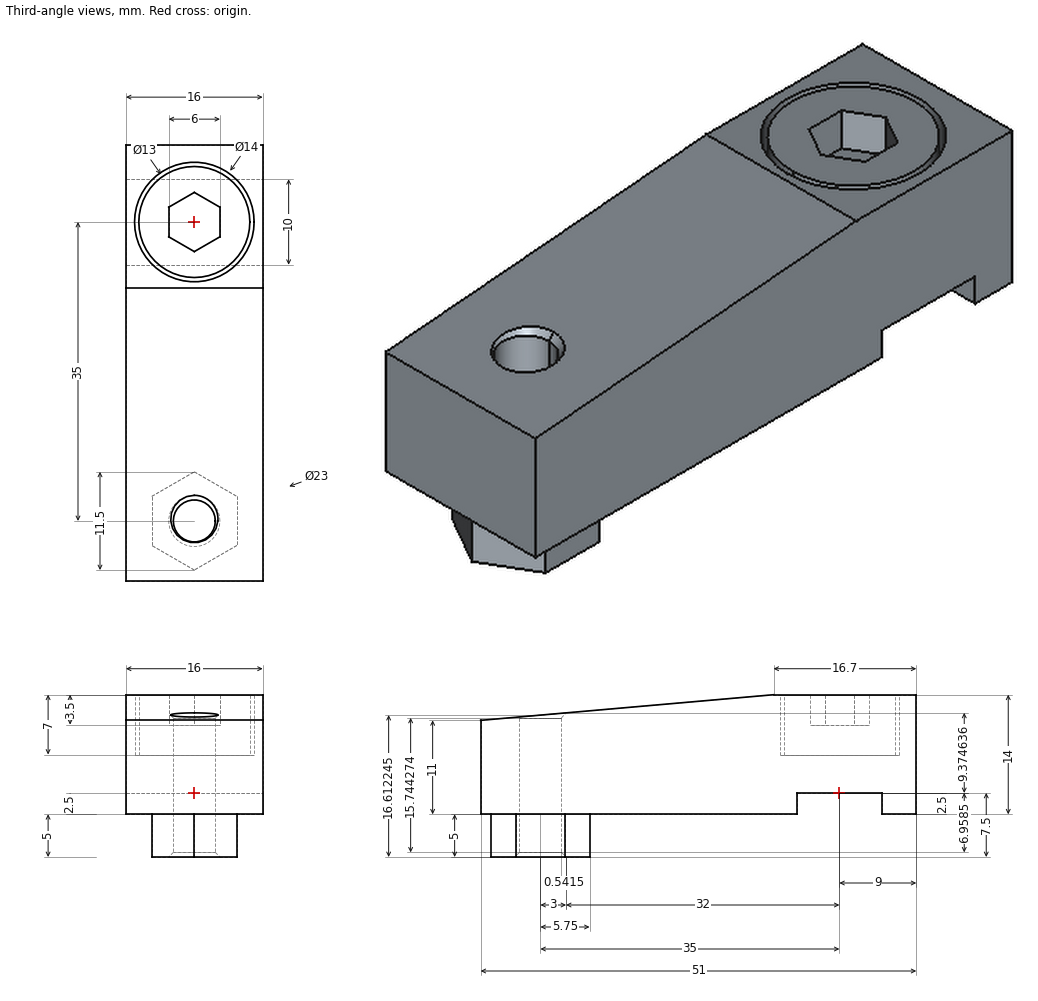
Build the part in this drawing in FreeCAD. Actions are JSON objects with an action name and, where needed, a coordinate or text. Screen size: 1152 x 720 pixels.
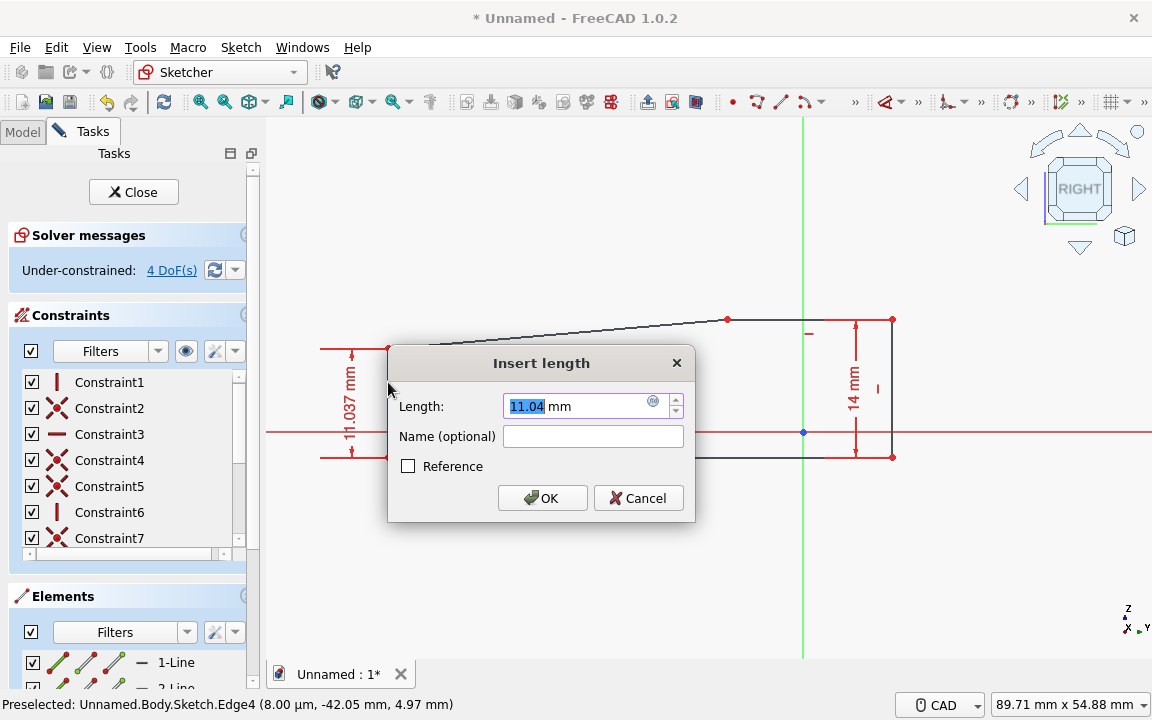
{"action": "type", "text": "11"}
{"action": "key", "text": "Return"}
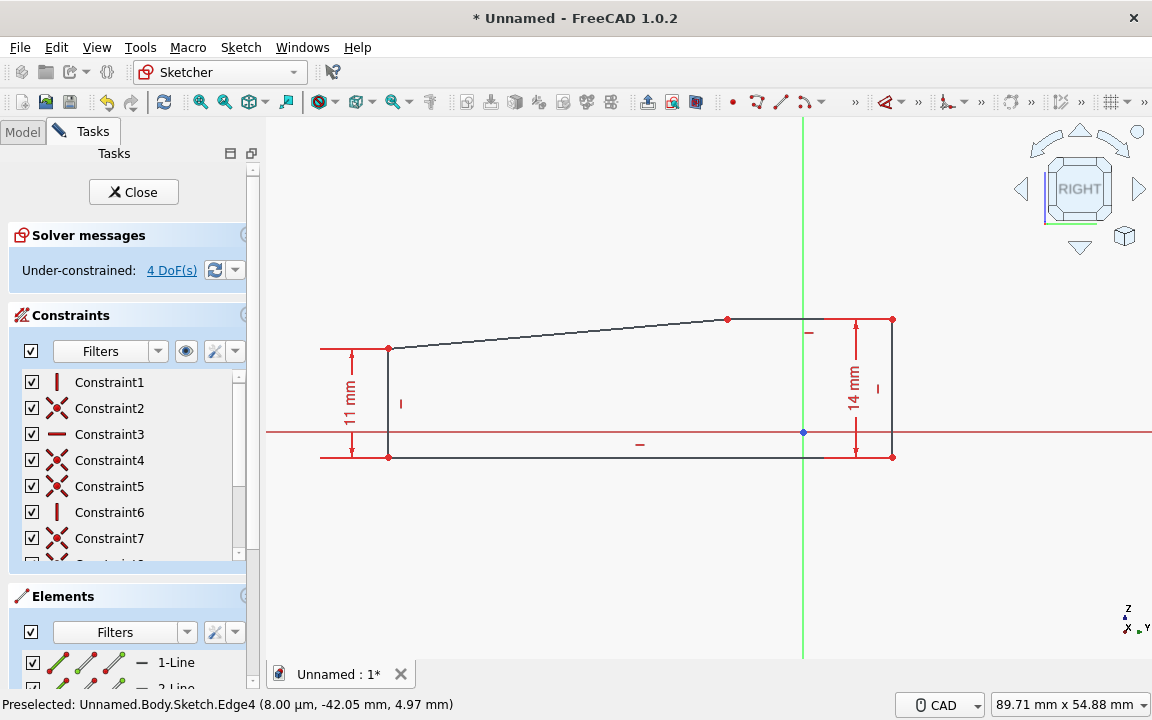
{"action": "left_click", "coordinate": [539, 458]}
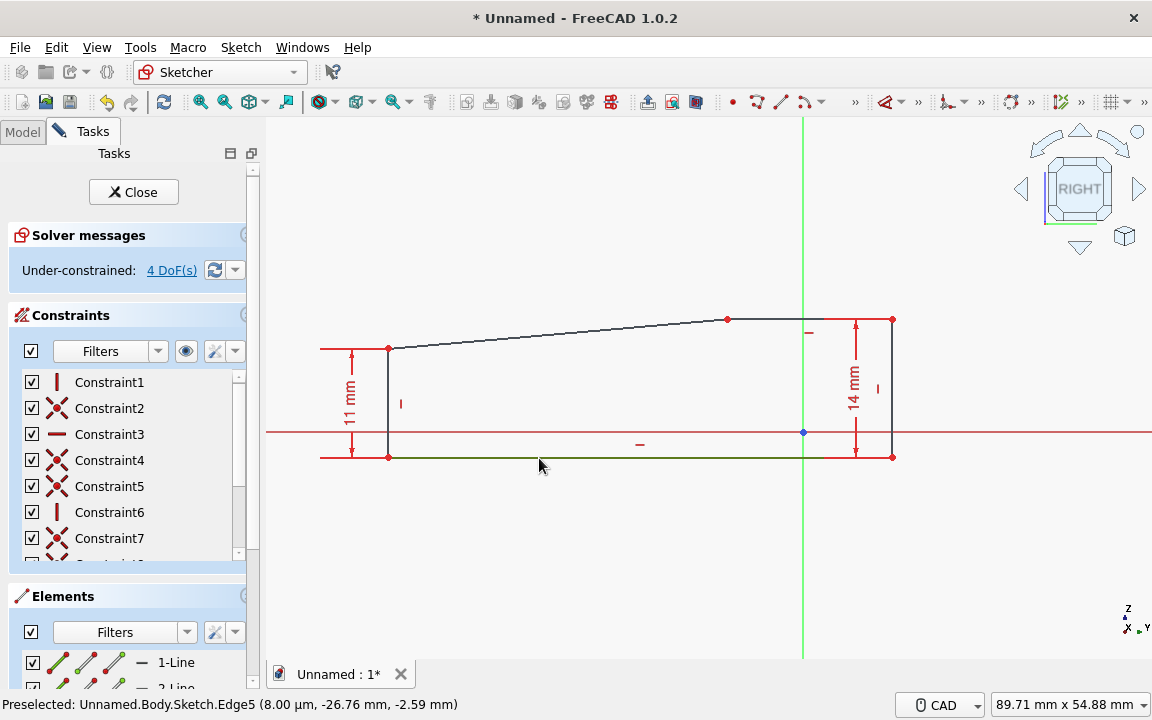
{"action": "left_click", "coordinate": [904, 102]}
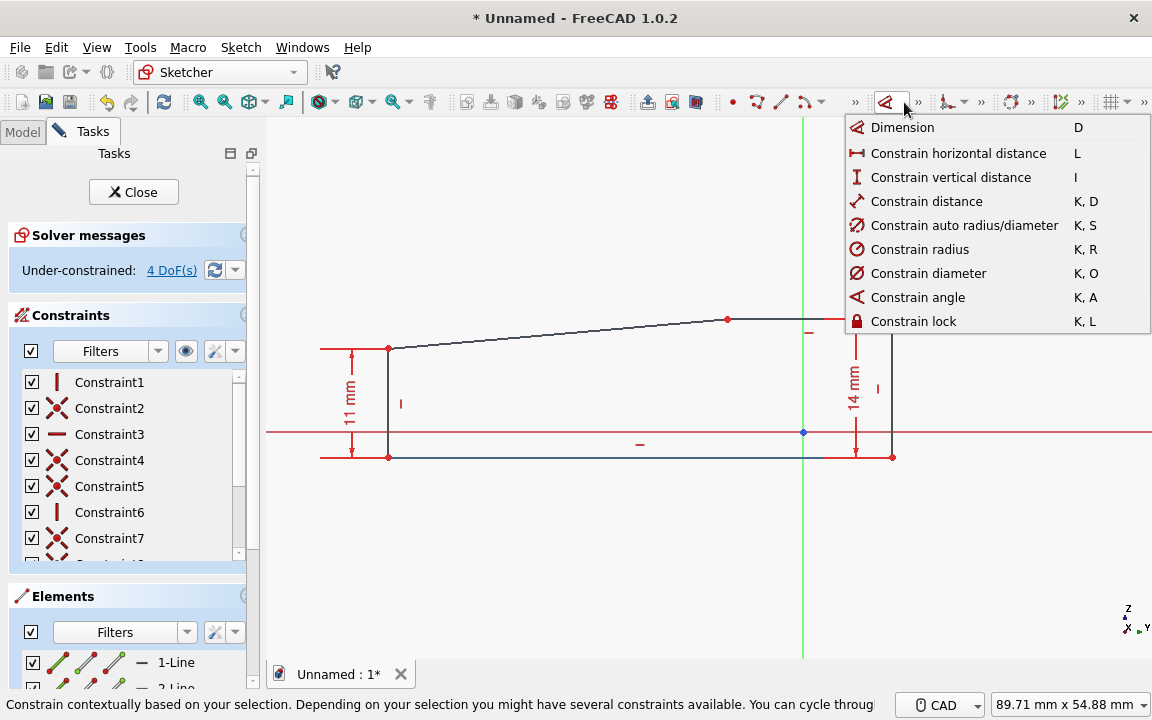
{"action": "left_click", "coordinate": [998, 153]}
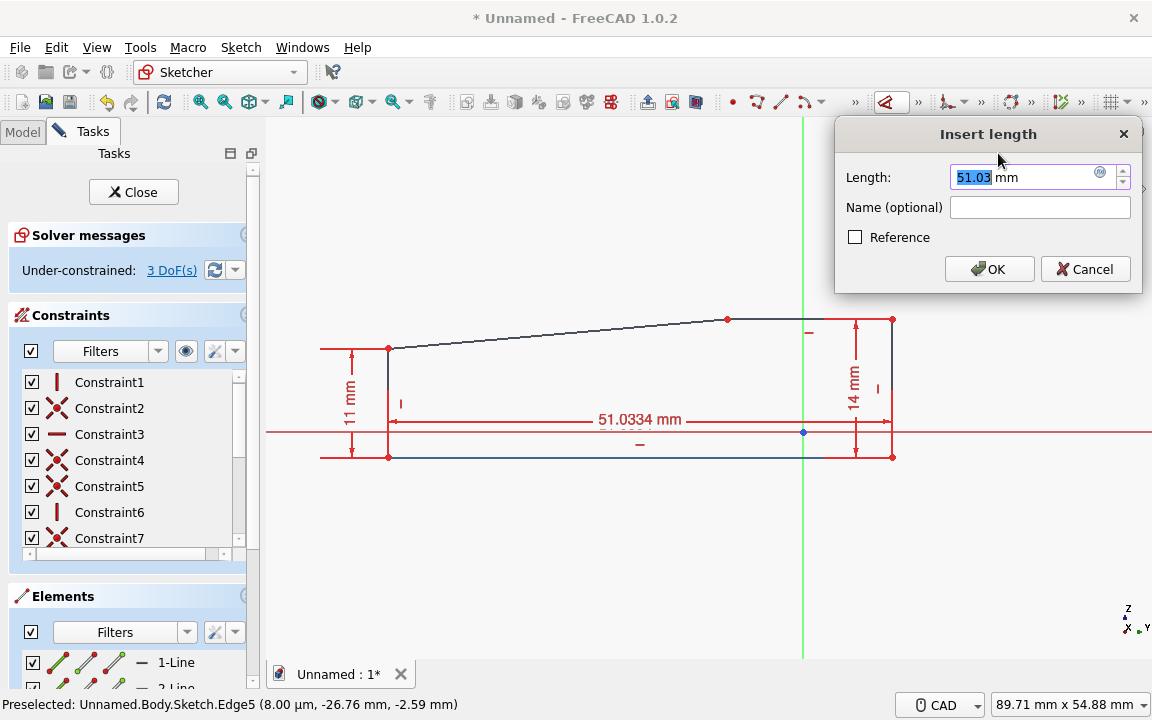
{"action": "type", "text": "51"}
{"action": "key", "text": "Return"}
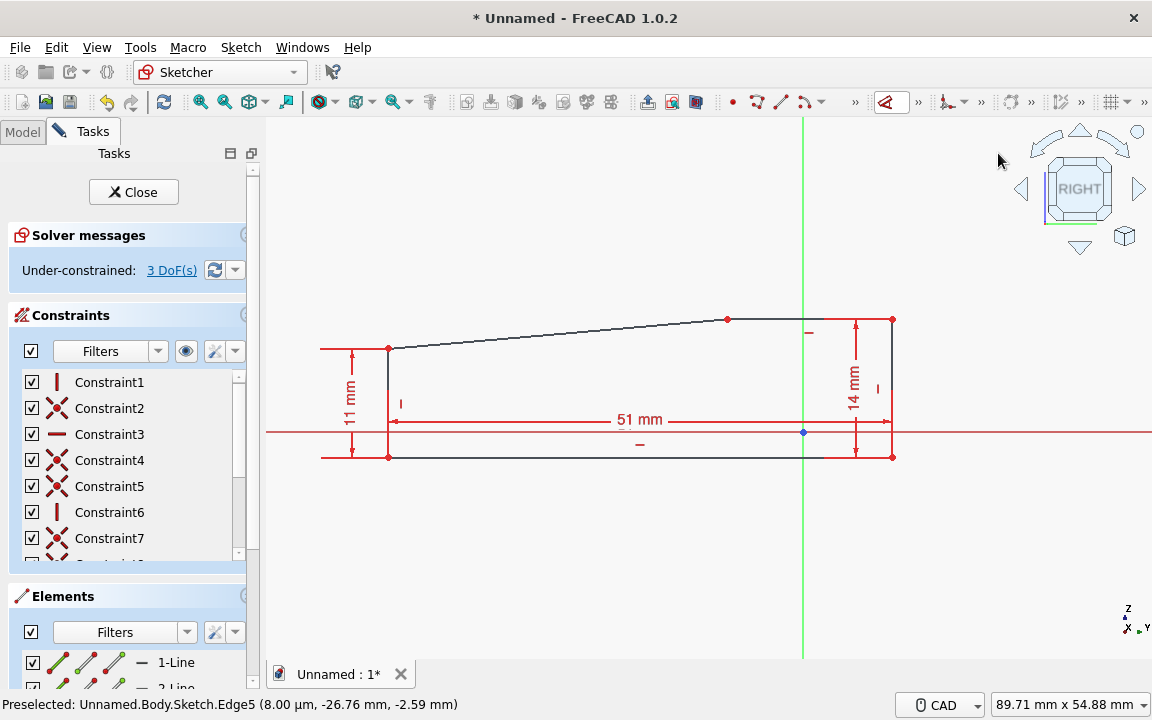
{"action": "left_click", "coordinate": [892, 458]}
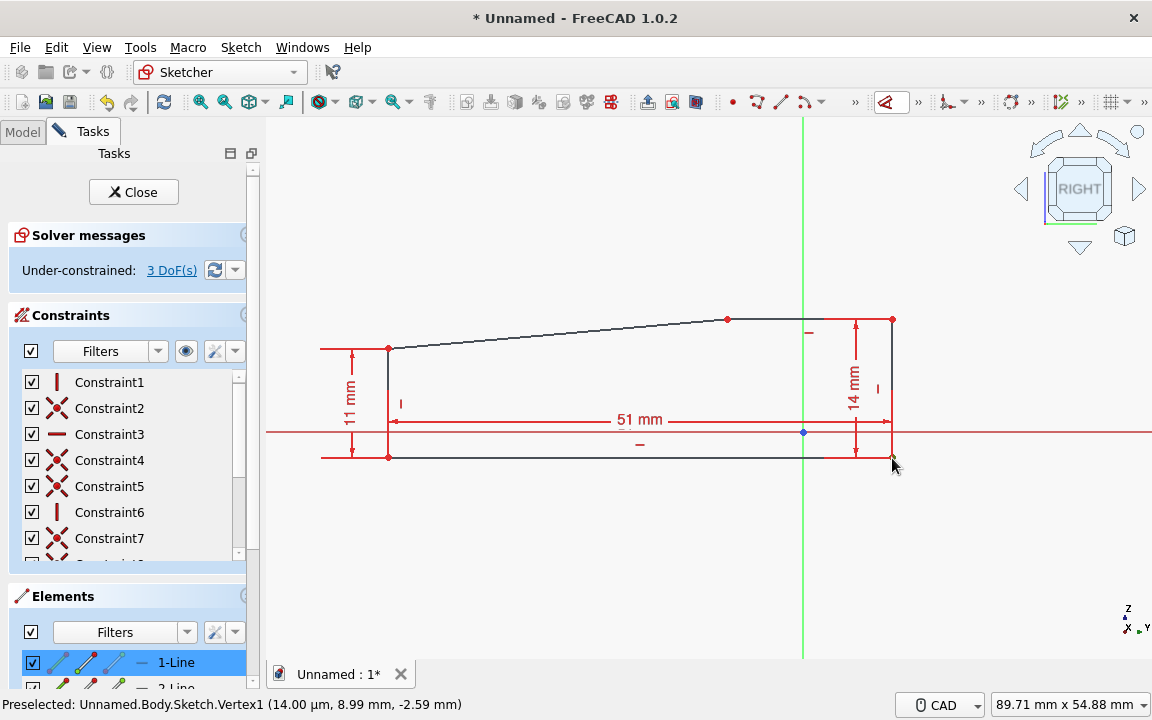
{"action": "key", "text": "l"}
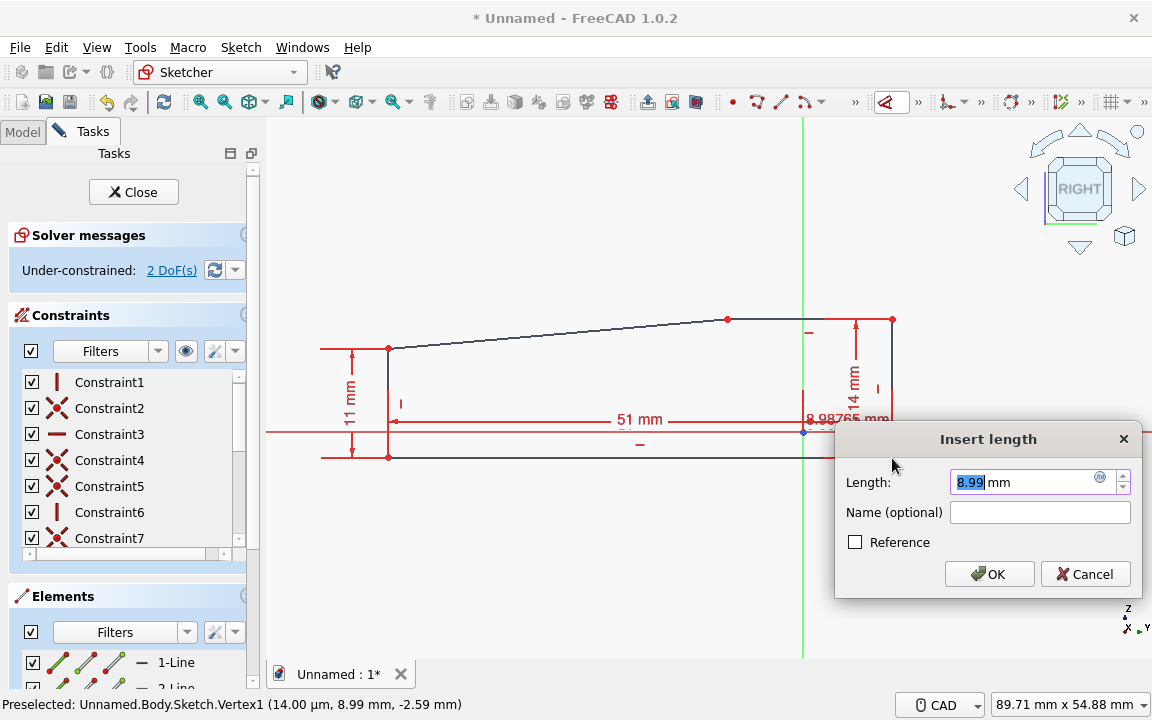
{"action": "type", "text": "9"}
{"action": "key", "text": "Return"}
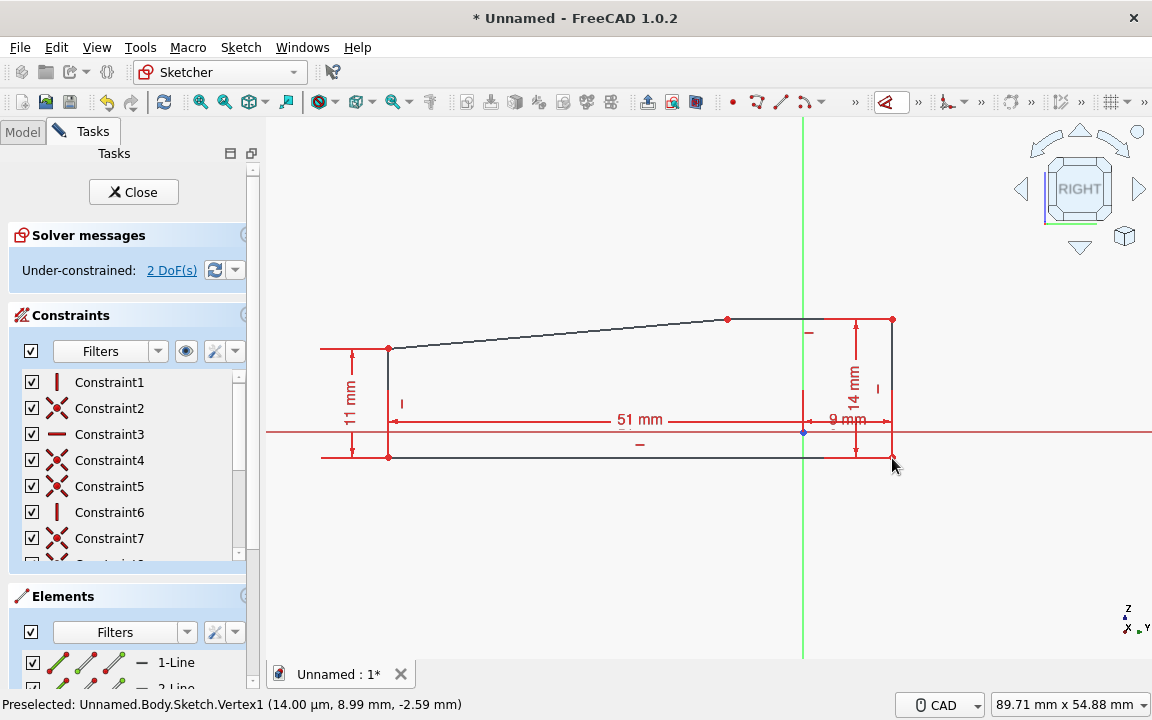
{"action": "left_click", "coordinate": [843, 319]}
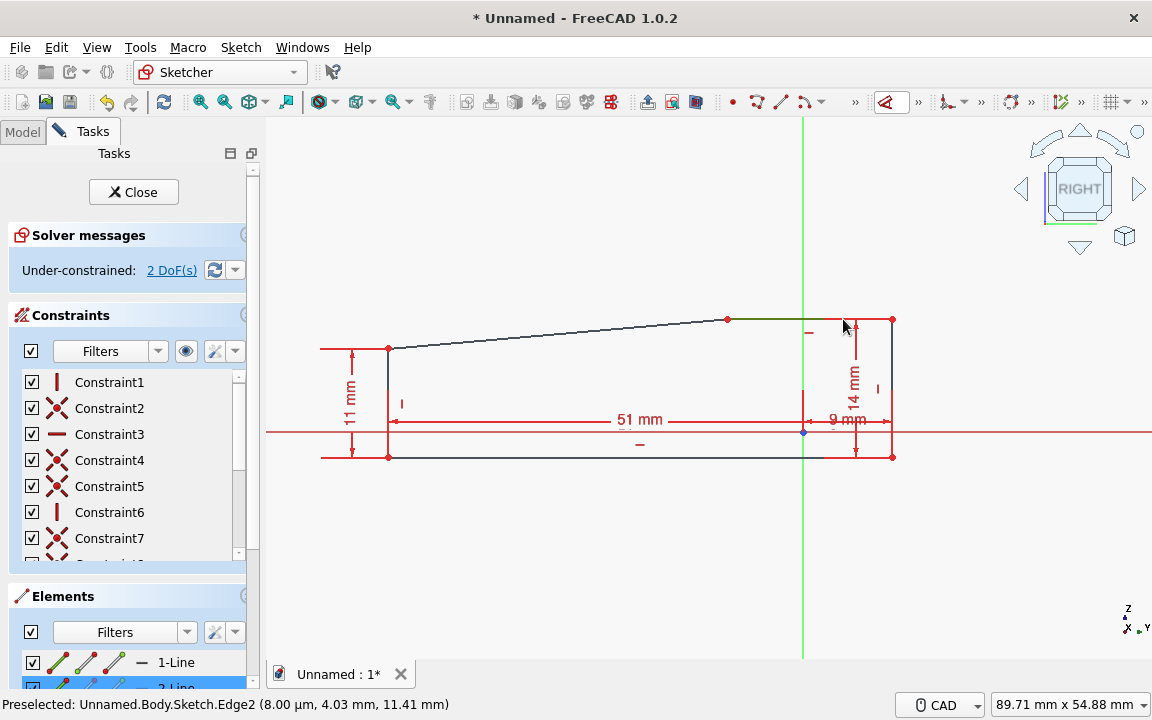
{"action": "left_click", "coordinate": [904, 102]}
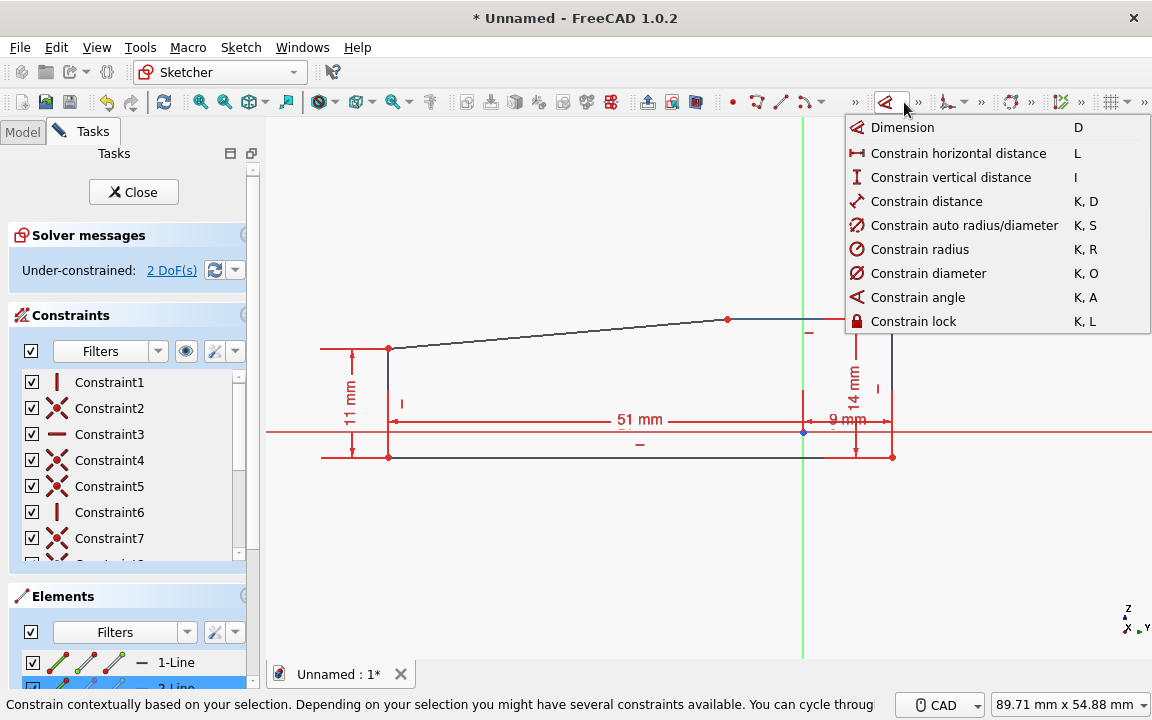
{"action": "left_click", "coordinate": [998, 153]}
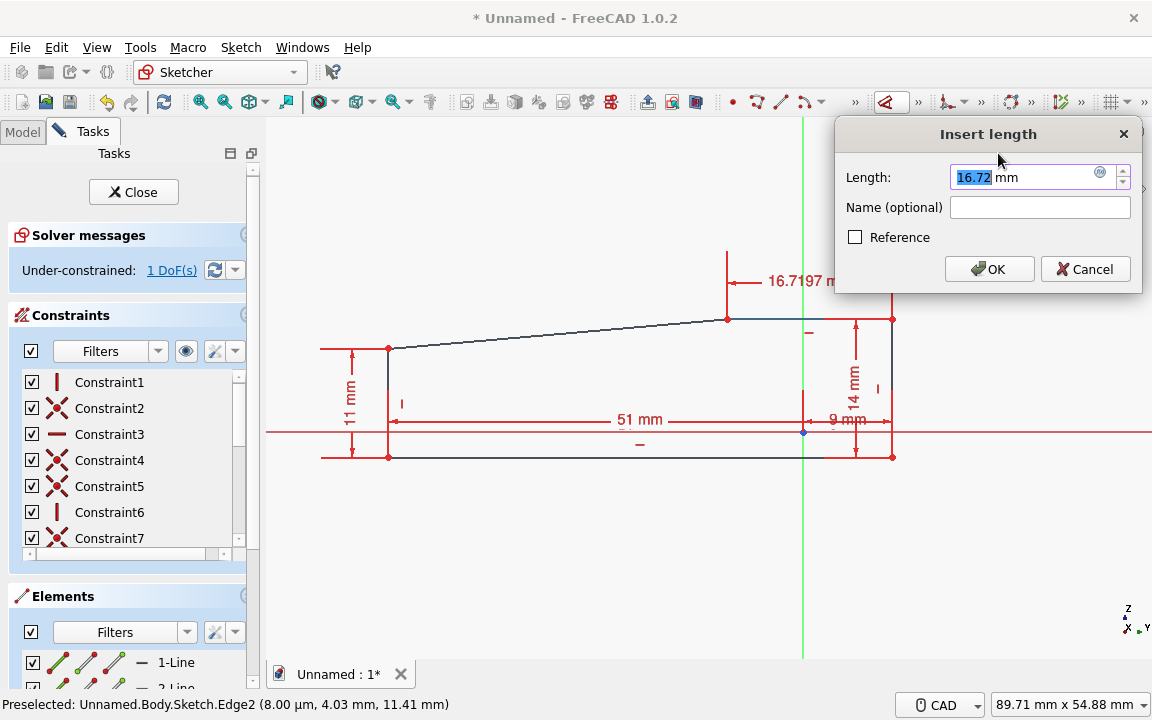
{"action": "type", "text": "16.7"}
{"action": "key", "text": "Return"}